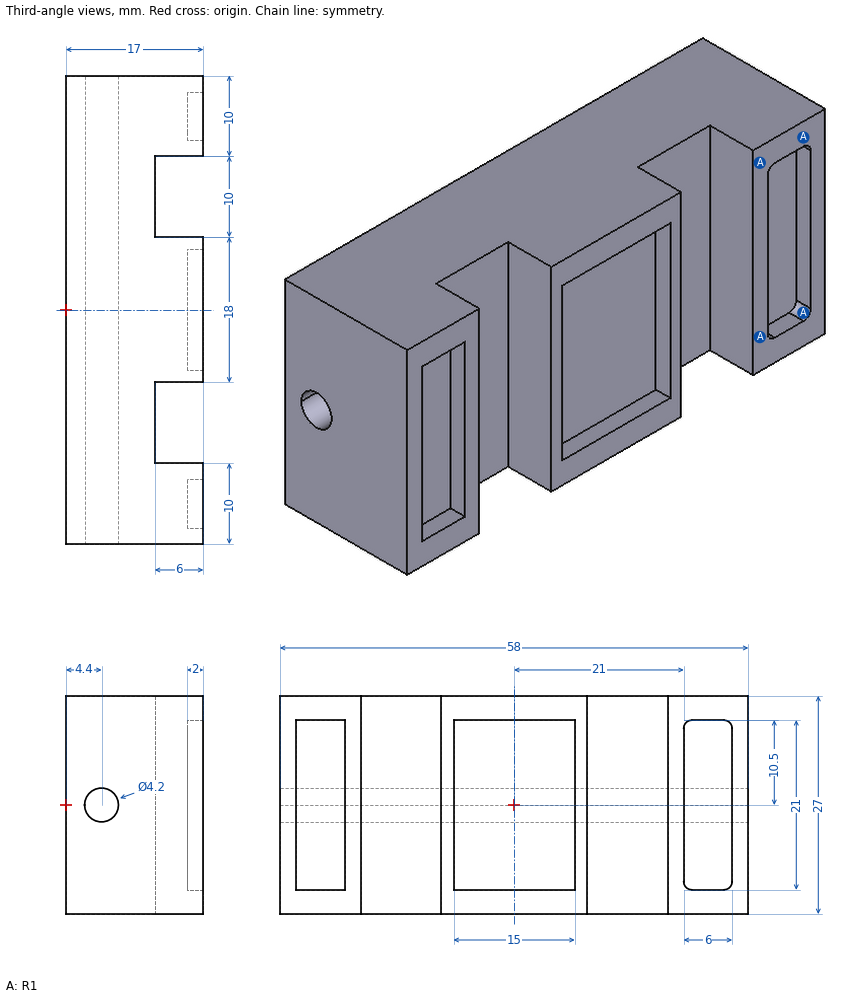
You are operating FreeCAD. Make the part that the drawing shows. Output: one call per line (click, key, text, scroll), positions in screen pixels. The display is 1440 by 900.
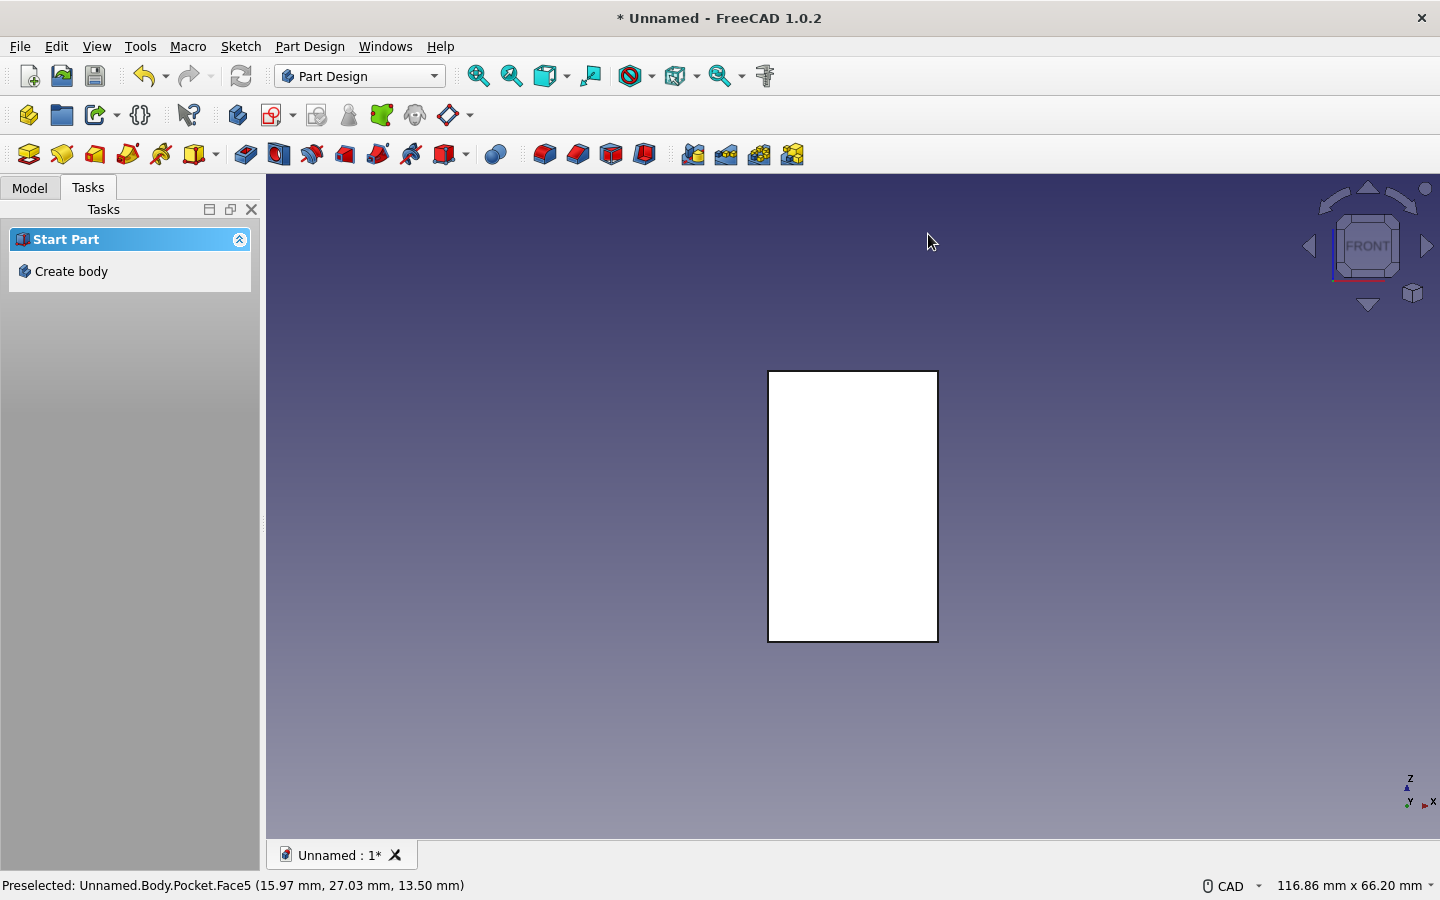
scroll(928, 611, up, 4)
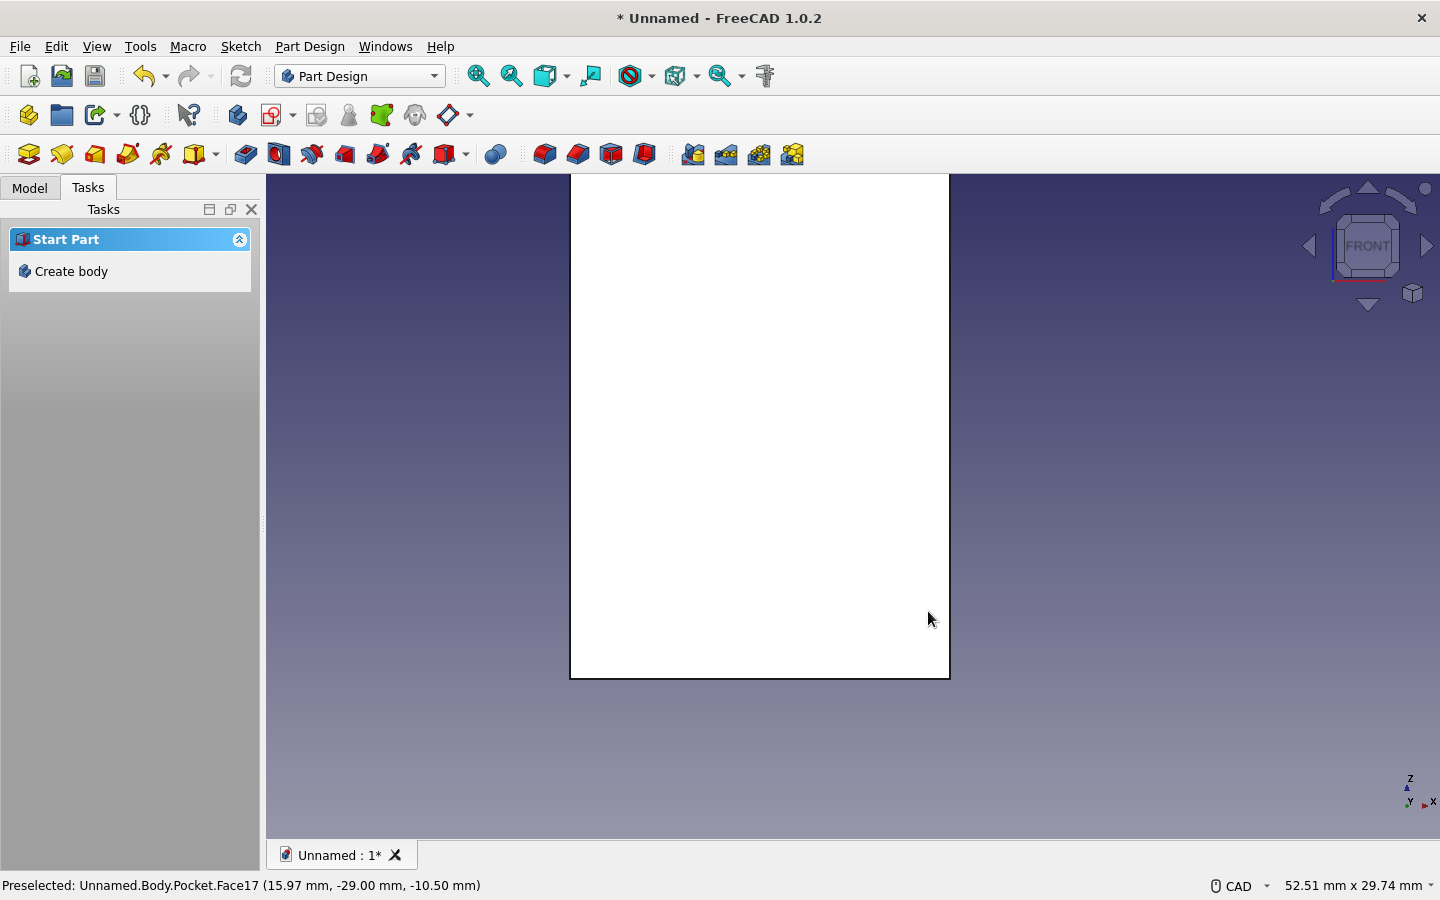
key(v)
key(f)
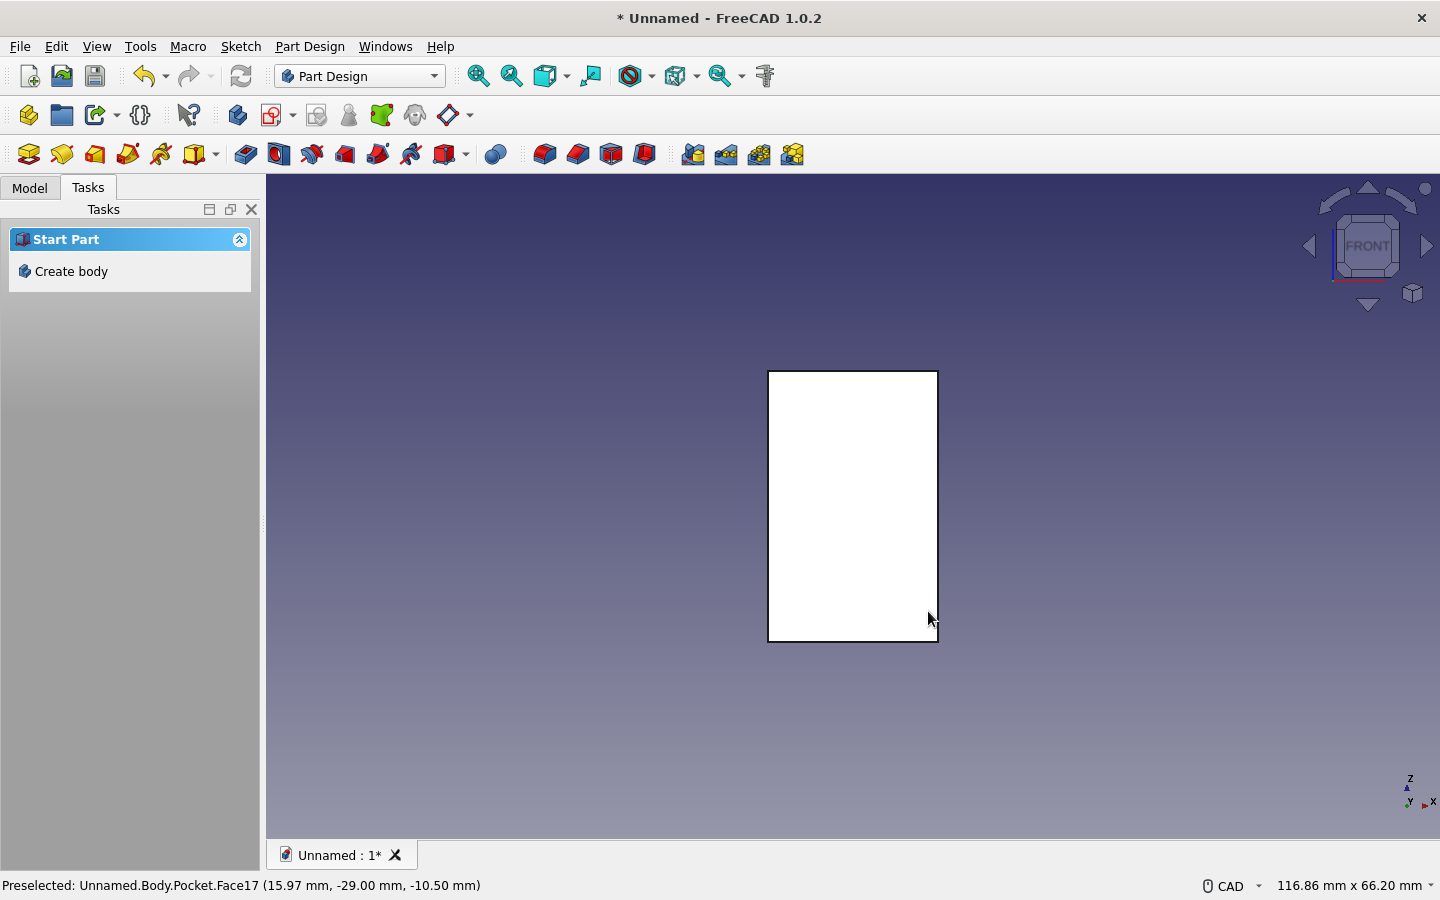
key(3)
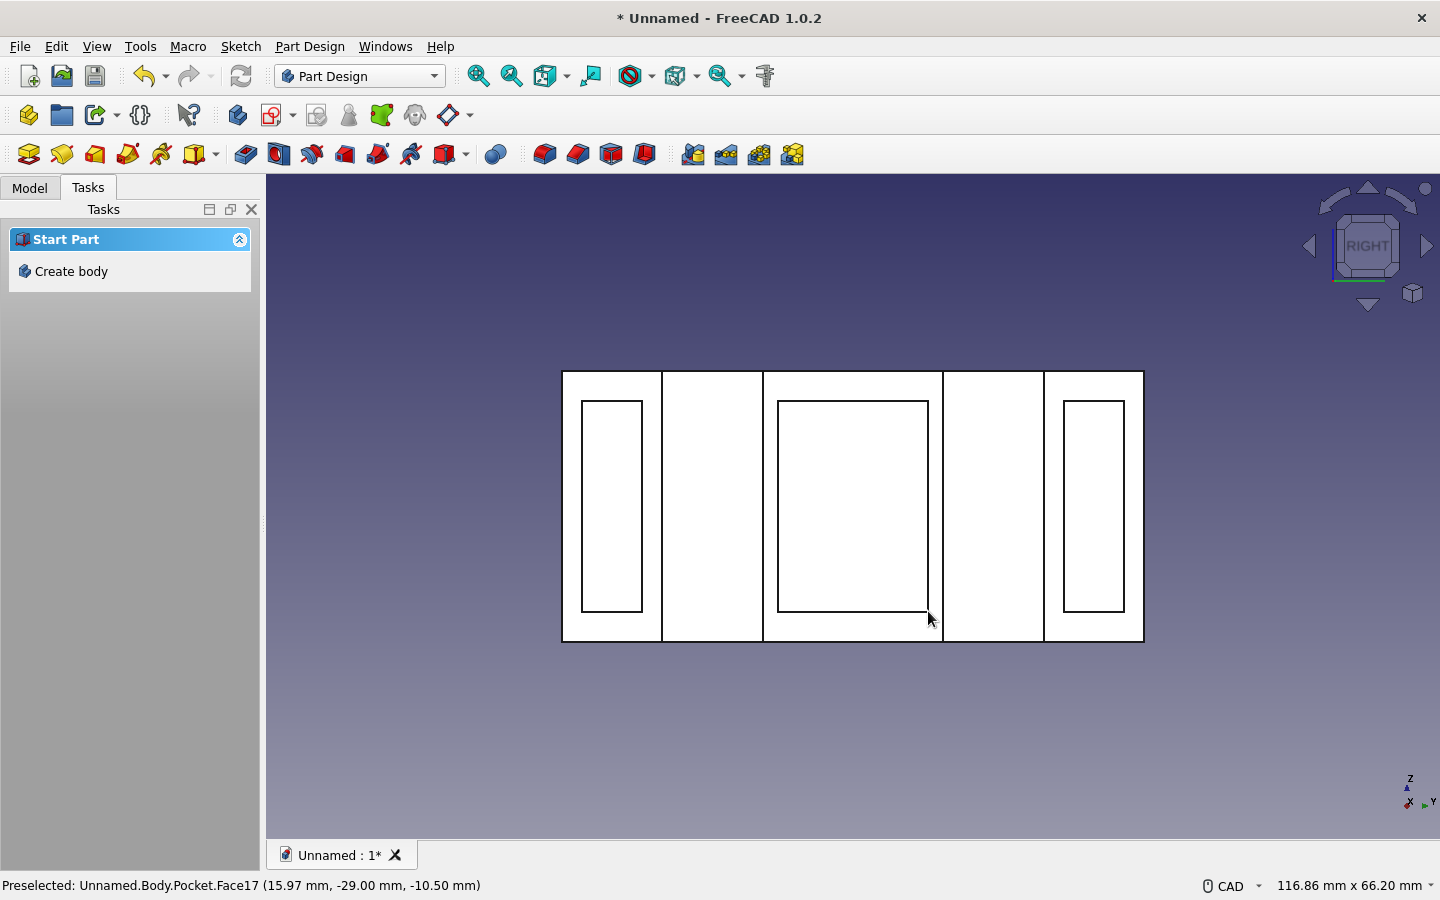
scroll(1124, 611, up, 4)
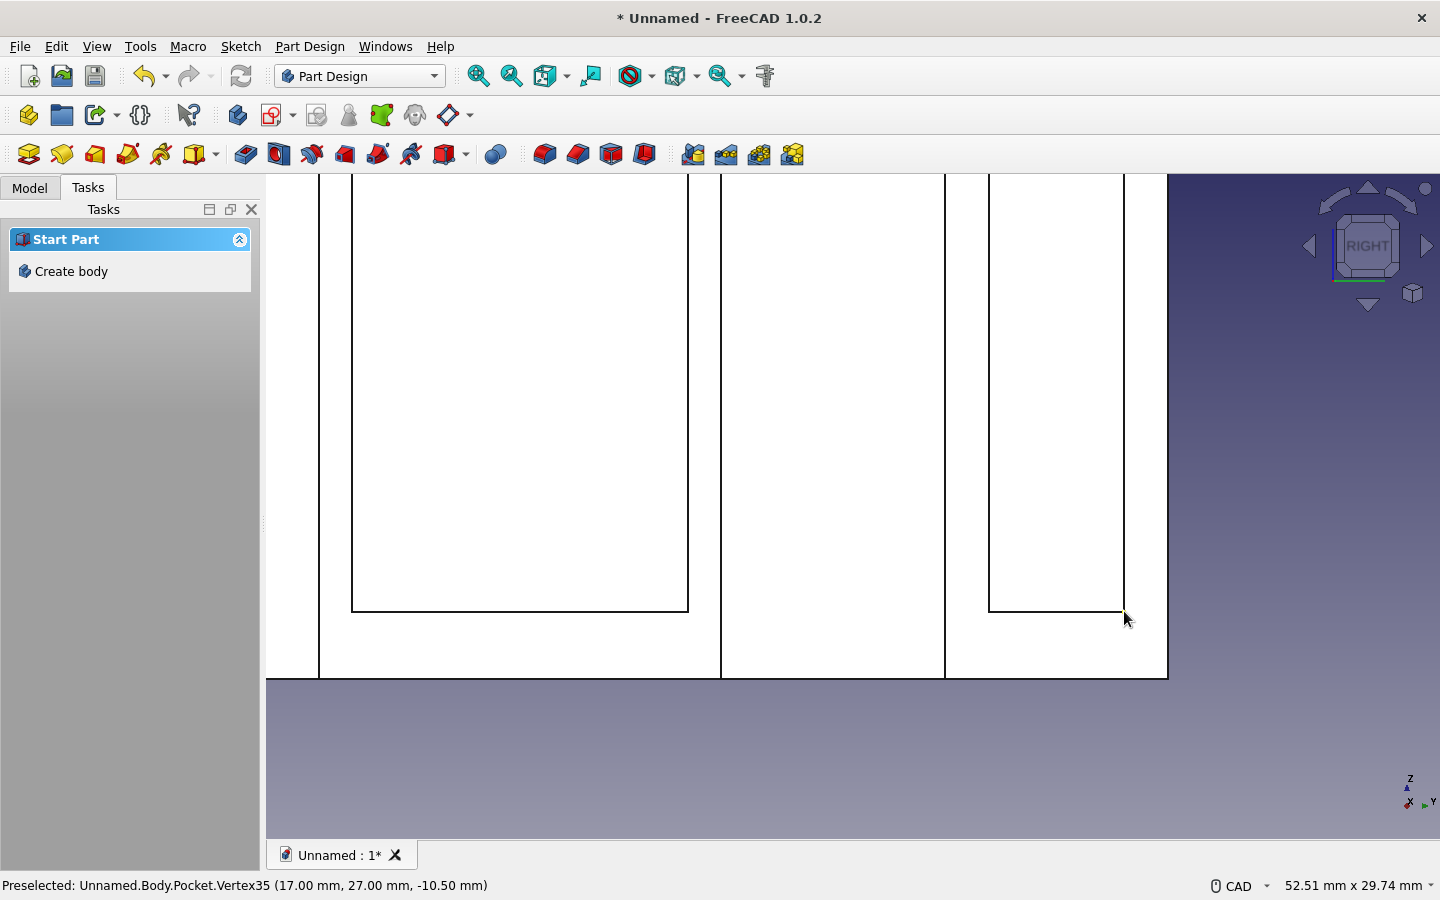
click(479, 76)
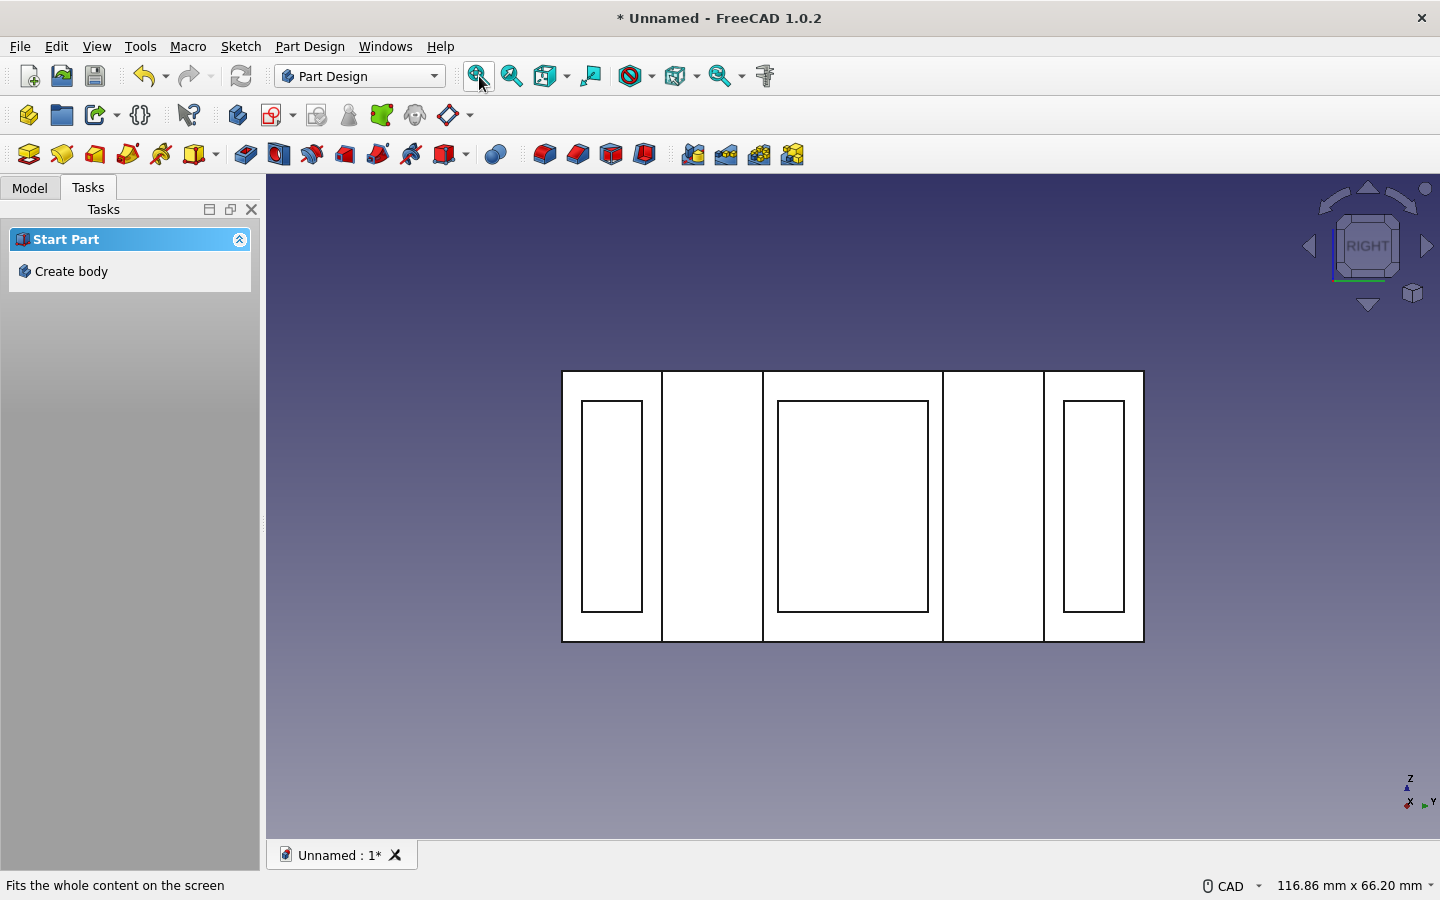
key(5)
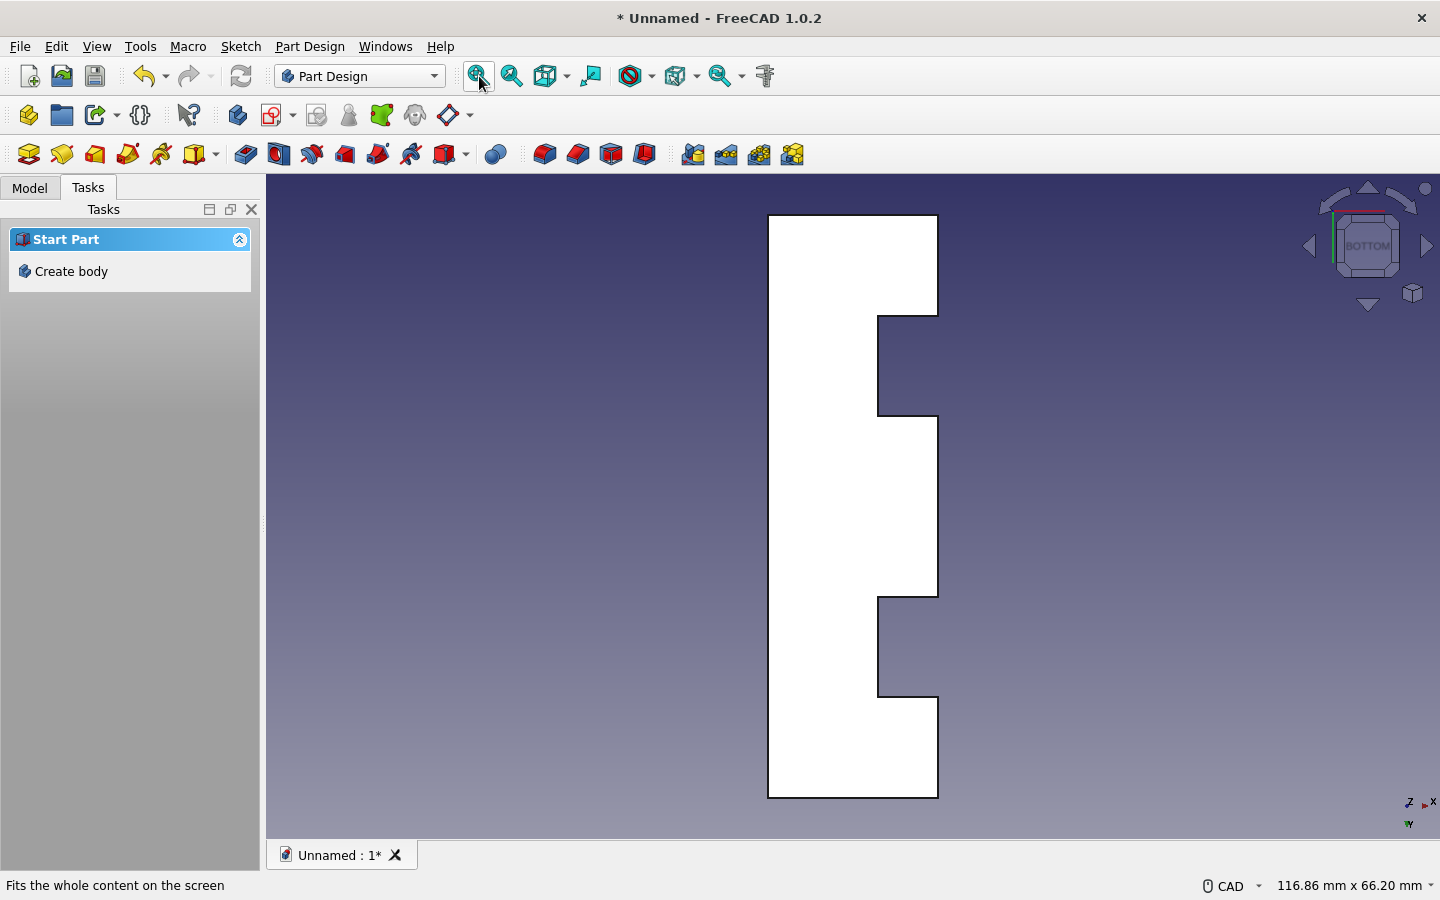
scroll(928, 777, up, 4)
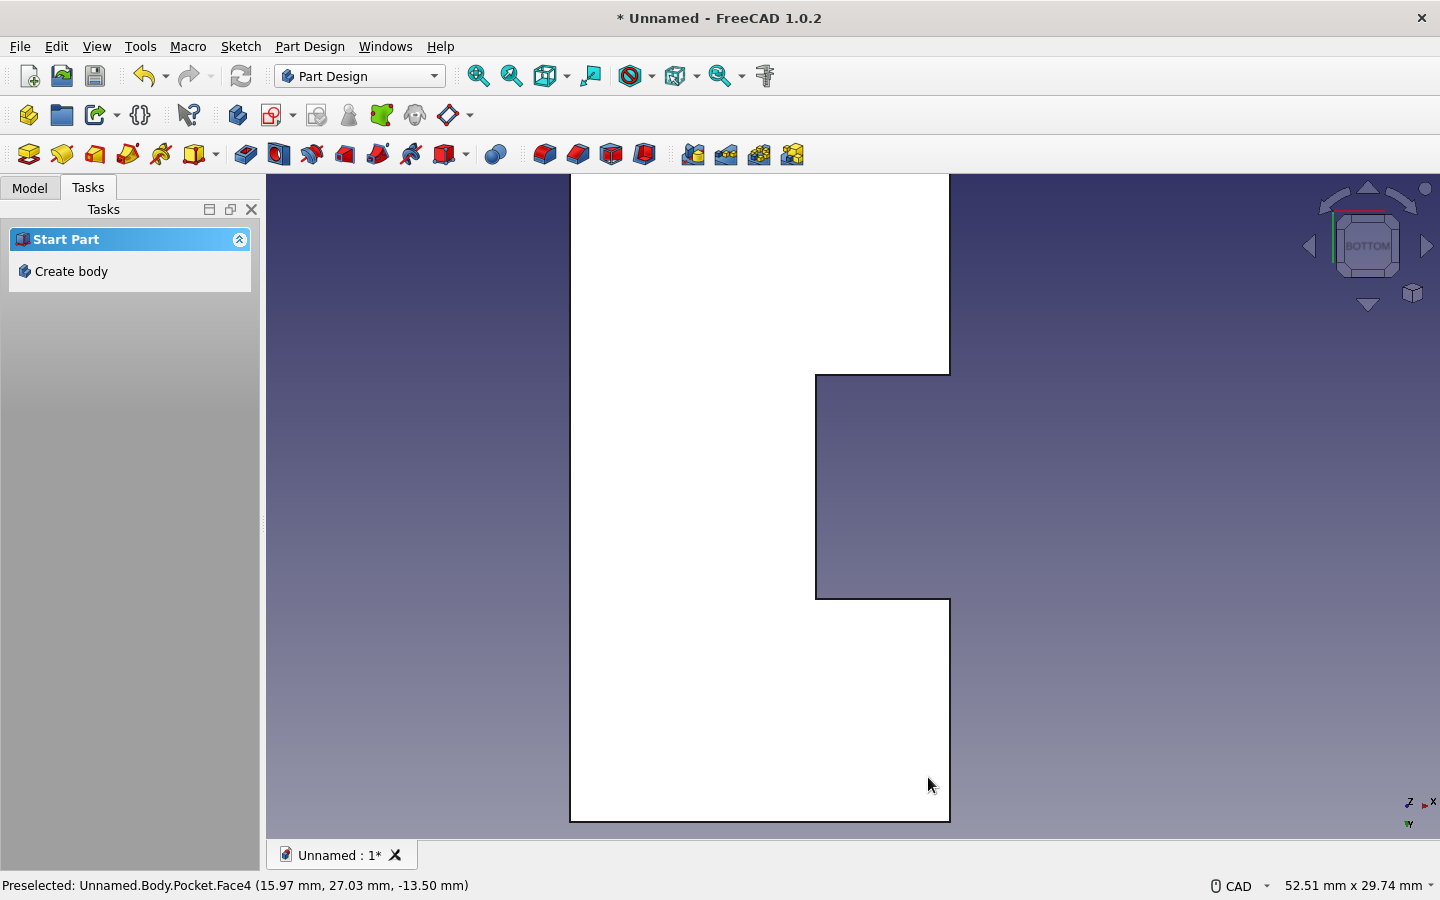
click(479, 76)